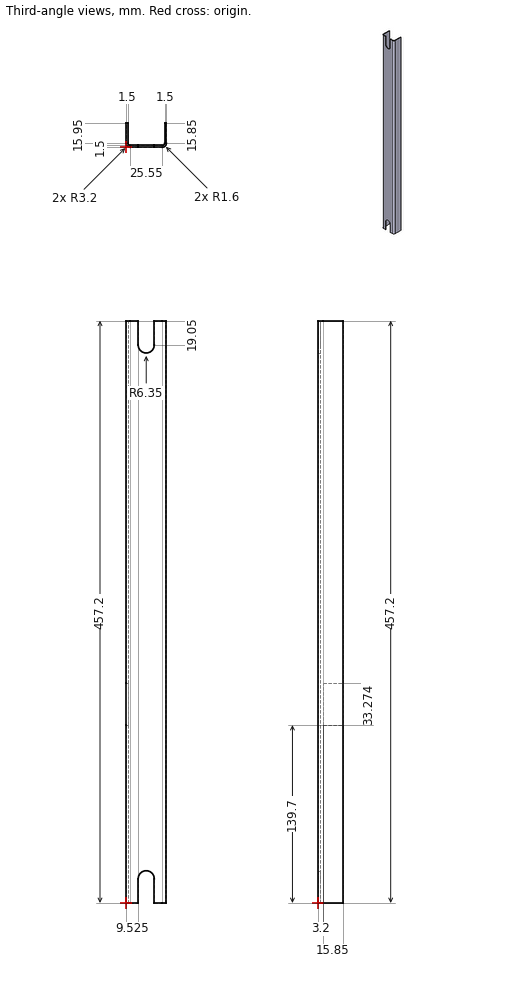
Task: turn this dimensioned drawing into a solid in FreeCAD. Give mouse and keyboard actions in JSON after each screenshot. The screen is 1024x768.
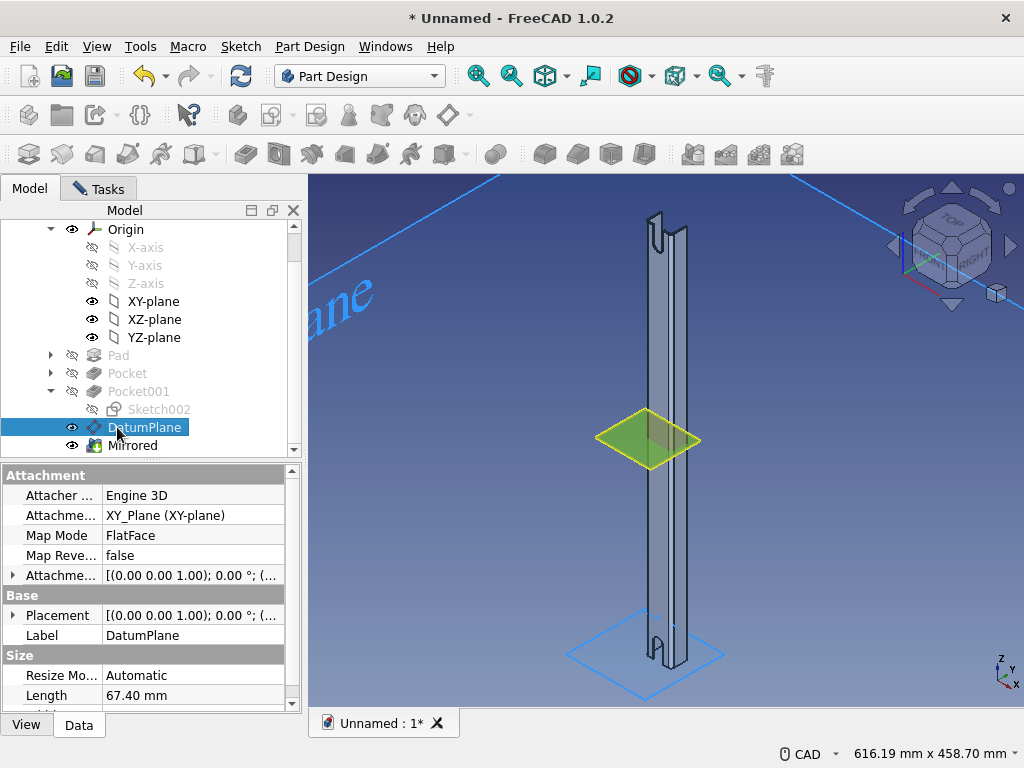
{"action": "left_click", "coordinate": [98, 188]}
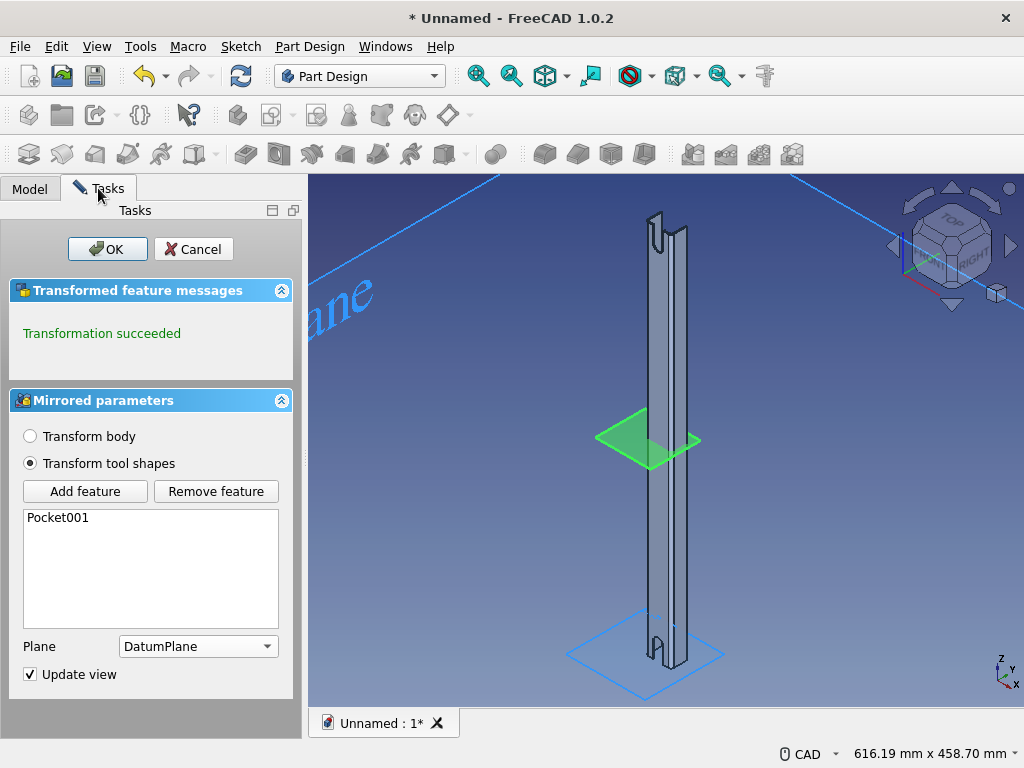
{"action": "left_click", "coordinate": [108, 249]}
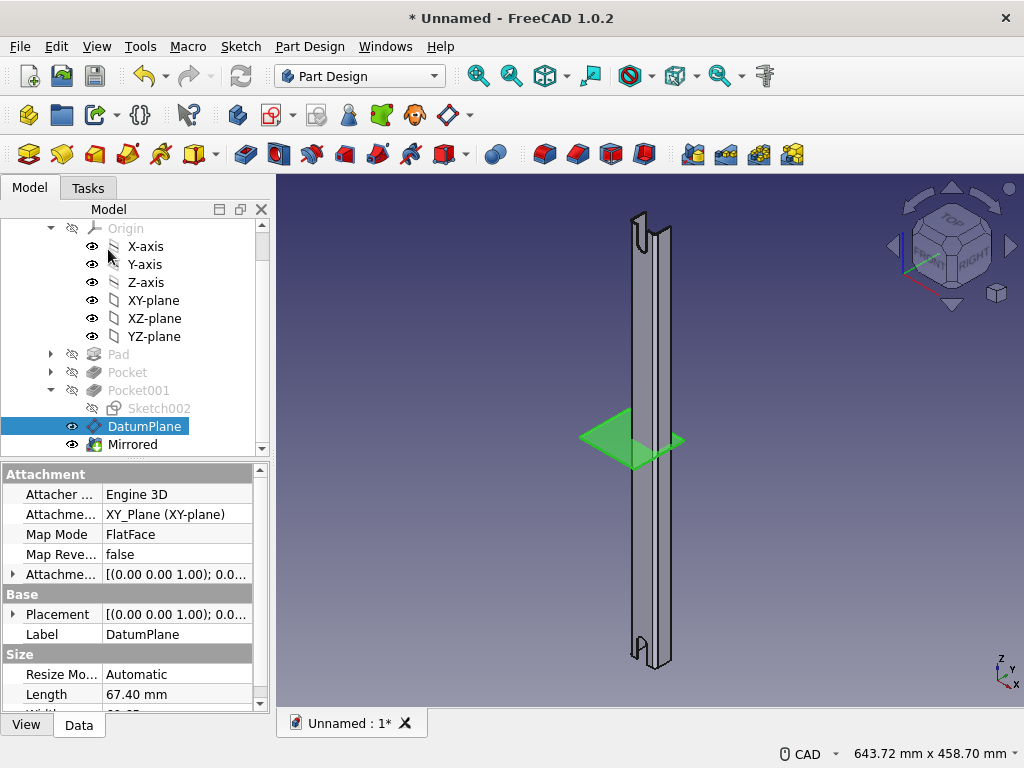
{"action": "left_click", "coordinate": [117, 426]}
{"action": "key", "text": "space"}